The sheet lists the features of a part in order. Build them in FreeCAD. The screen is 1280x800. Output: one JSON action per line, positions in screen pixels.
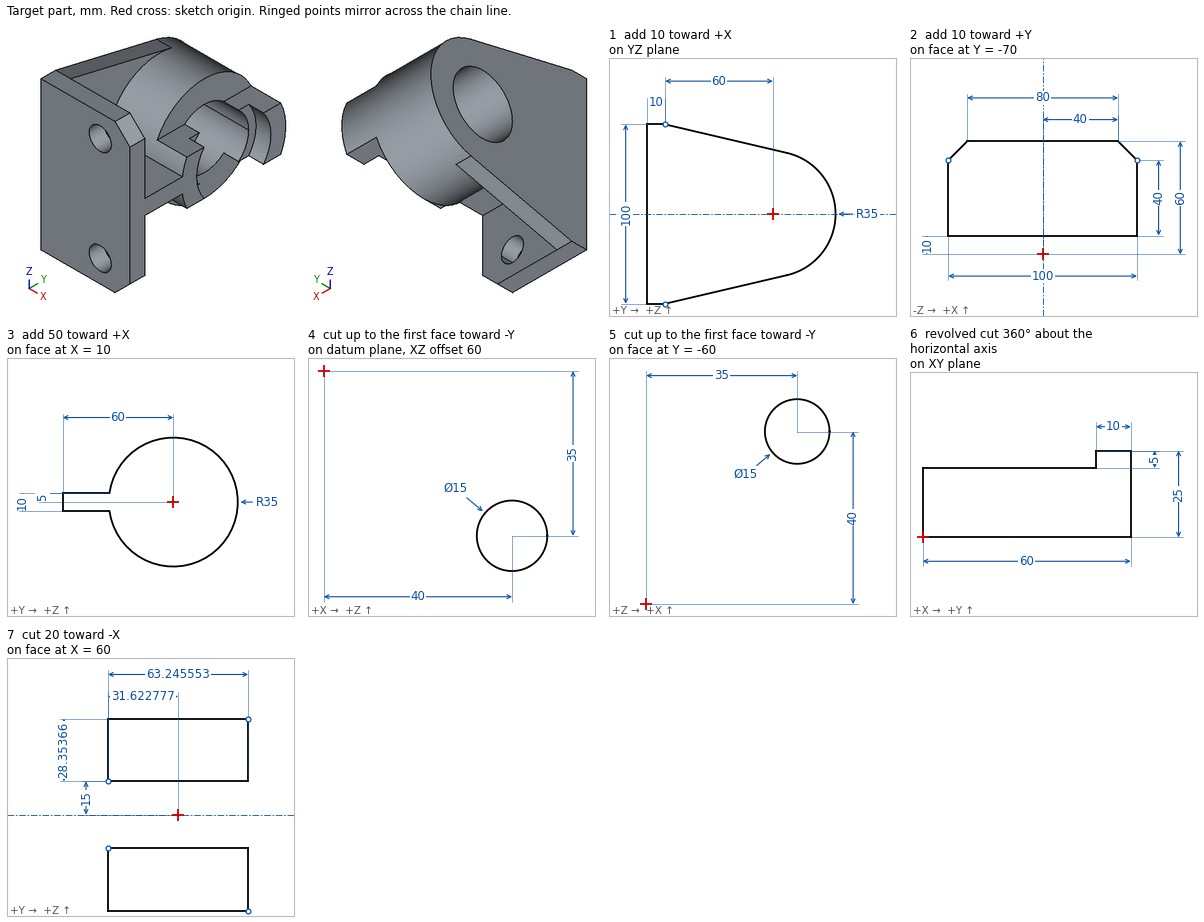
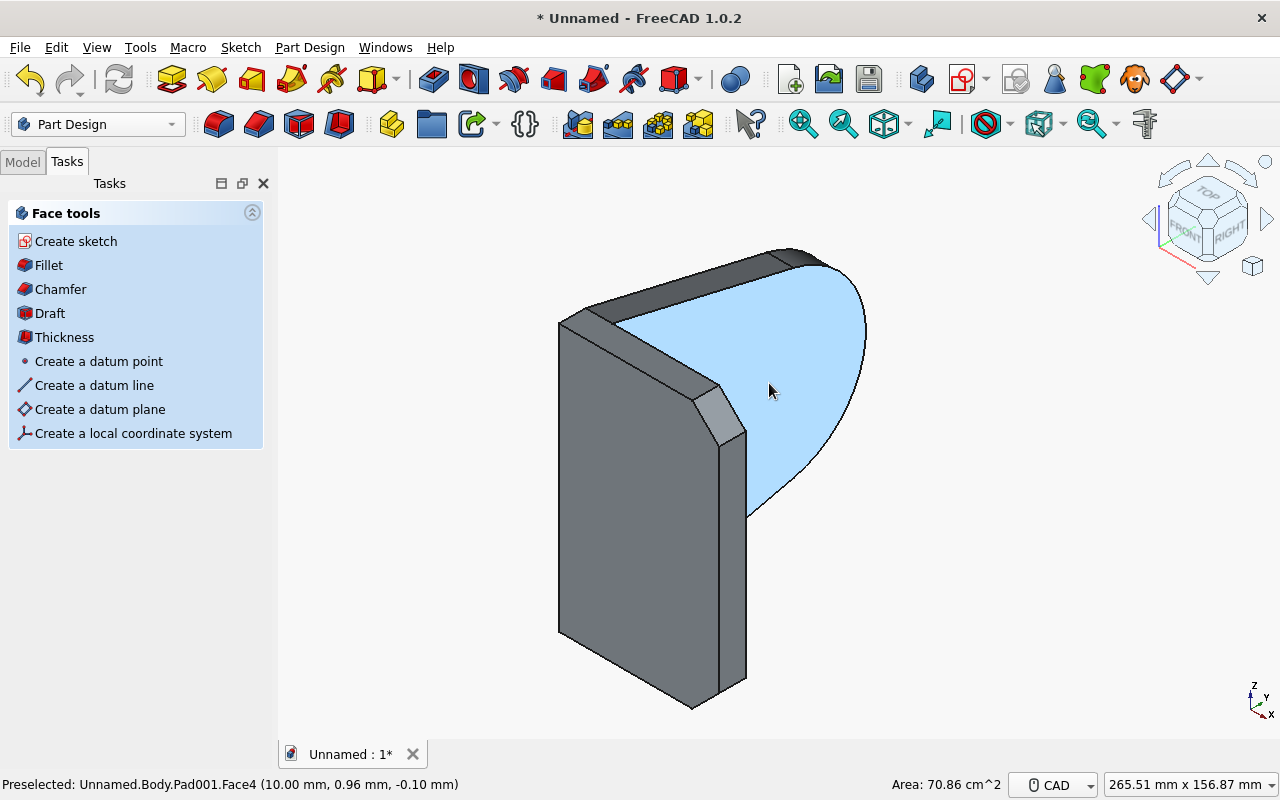
{"action": "left_click", "coordinate": [962, 80]}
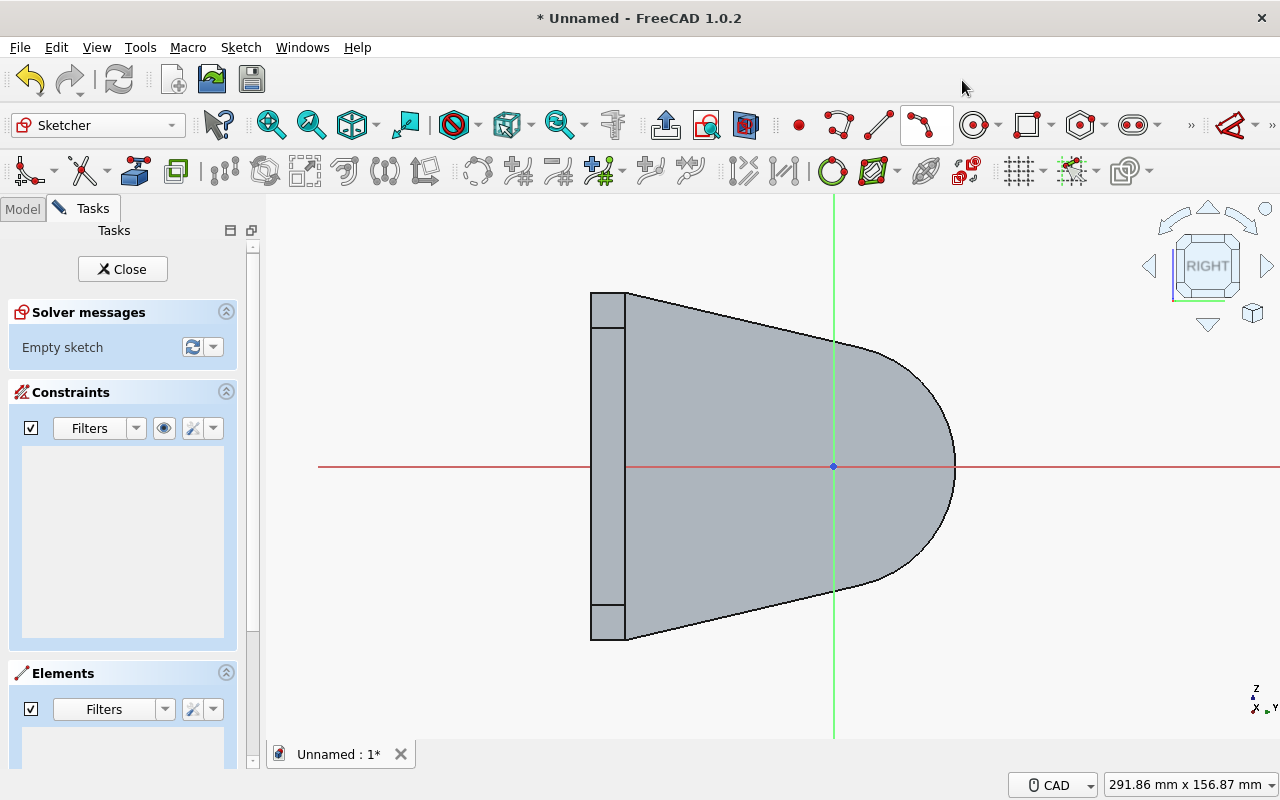
{"action": "left_click", "coordinate": [746, 126]}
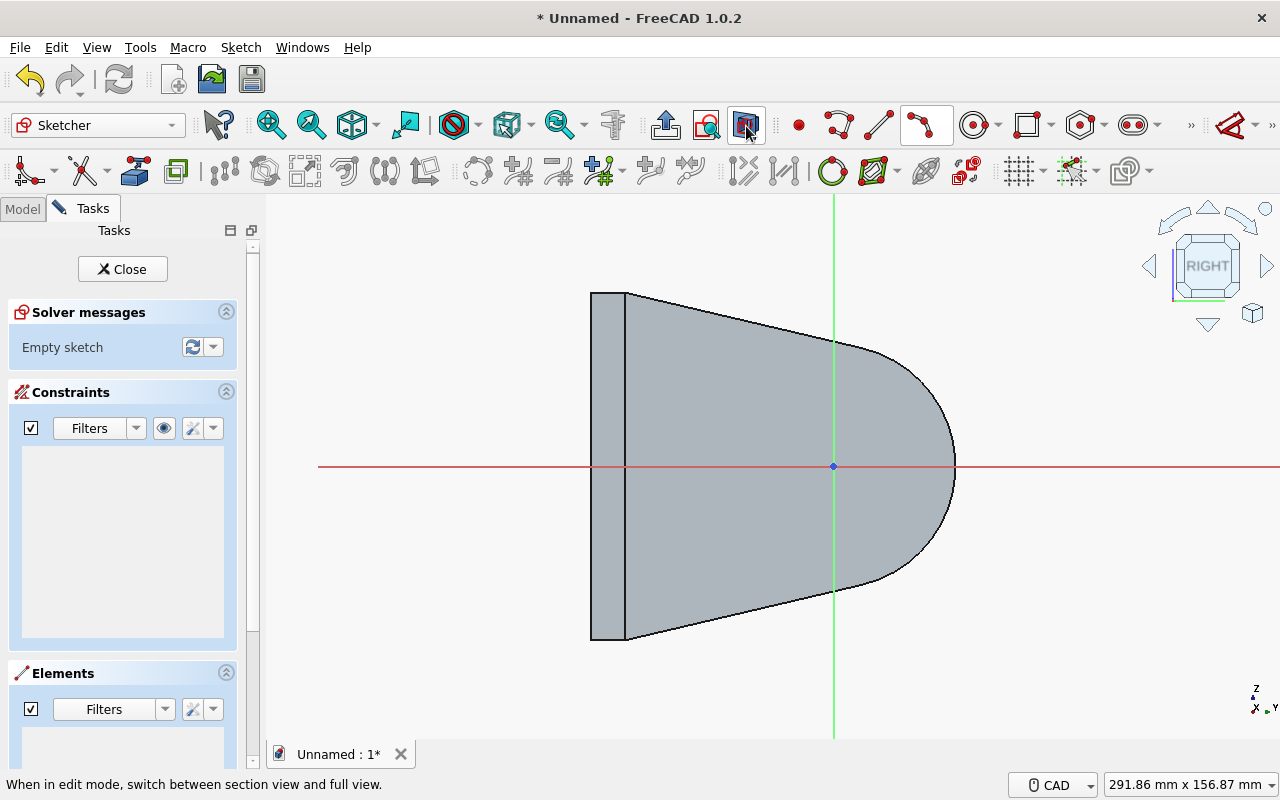
{"action": "scroll", "coordinate": [895, 466], "scroll_direction": "up", "scroll_amount": 3}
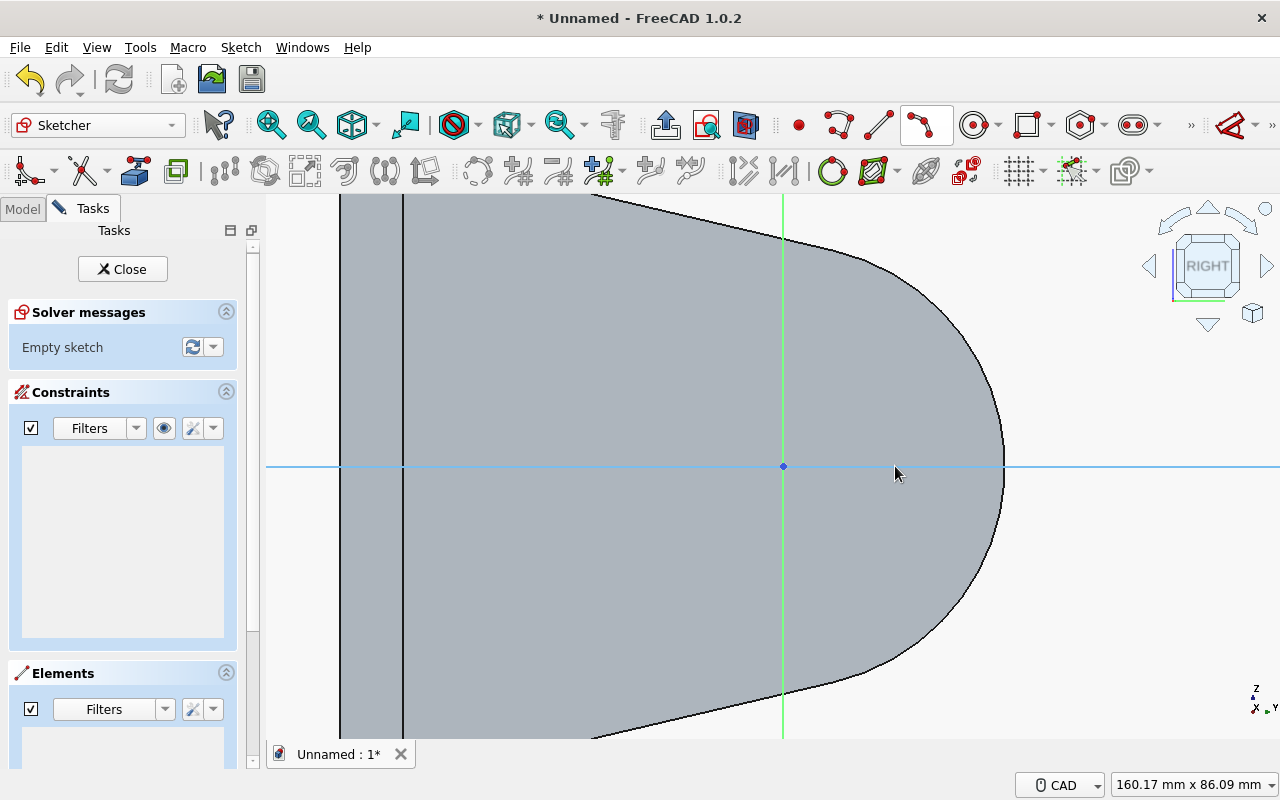
{"action": "left_click", "coordinate": [840, 126]}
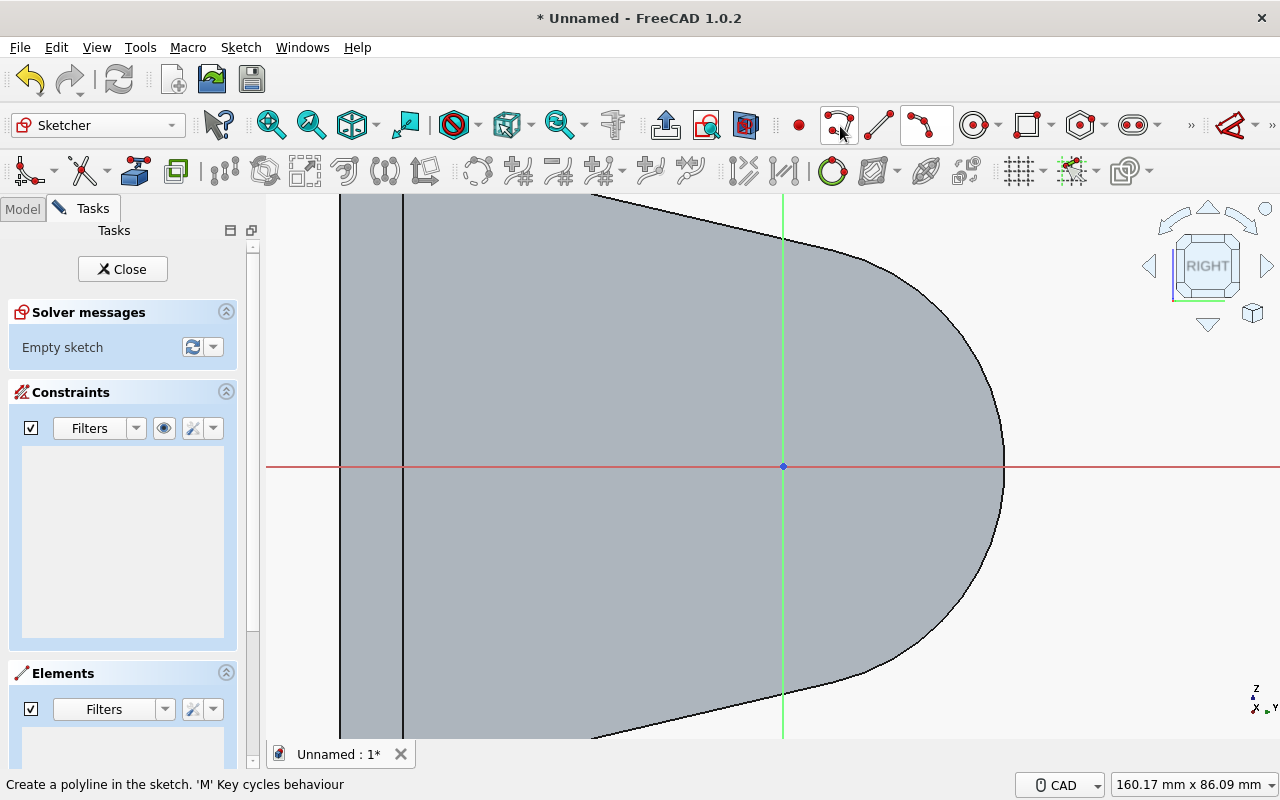
{"action": "left_click", "coordinate": [564, 435]}
{"action": "left_click", "coordinate": [403, 435]}
{"action": "left_click", "coordinate": [403, 498]}
{"action": "left_click", "coordinate": [564, 498]}
{"action": "right_click", "coordinate": [564, 498]}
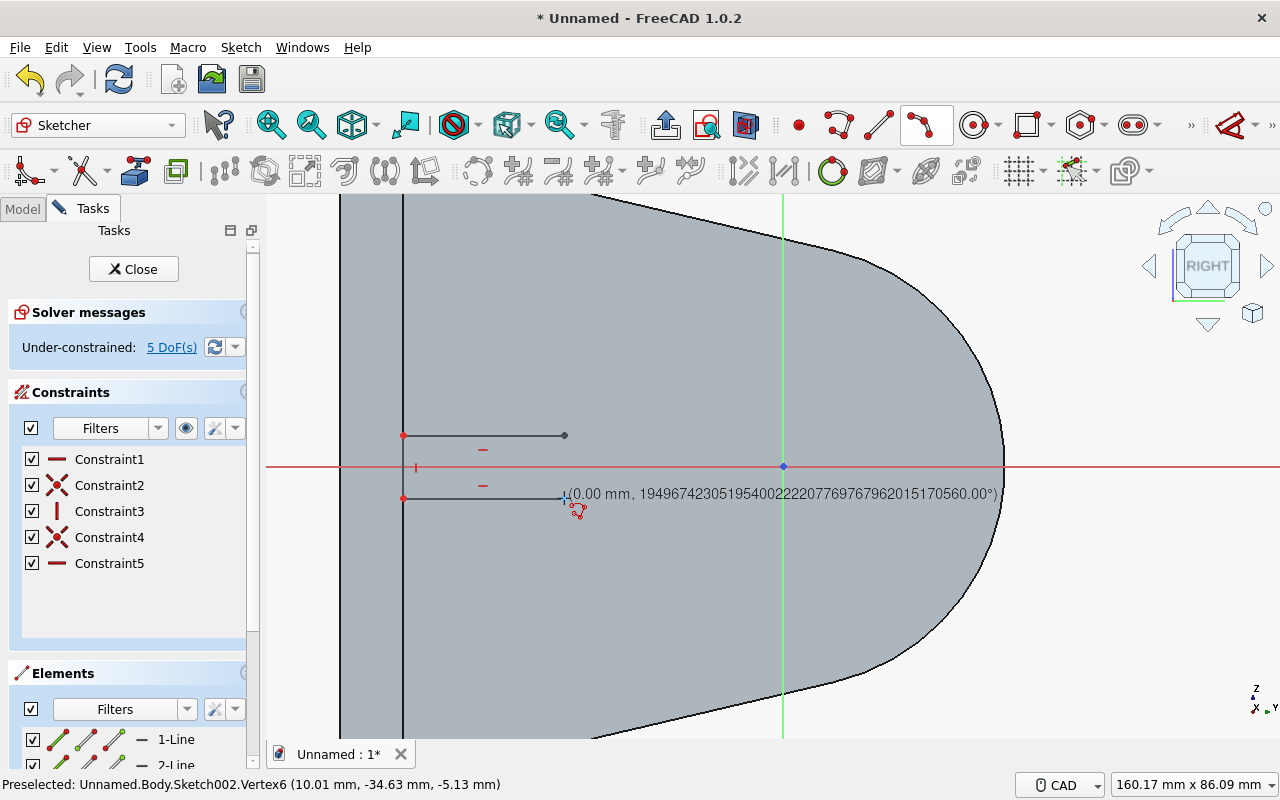
{"action": "left_click", "coordinate": [920, 126]}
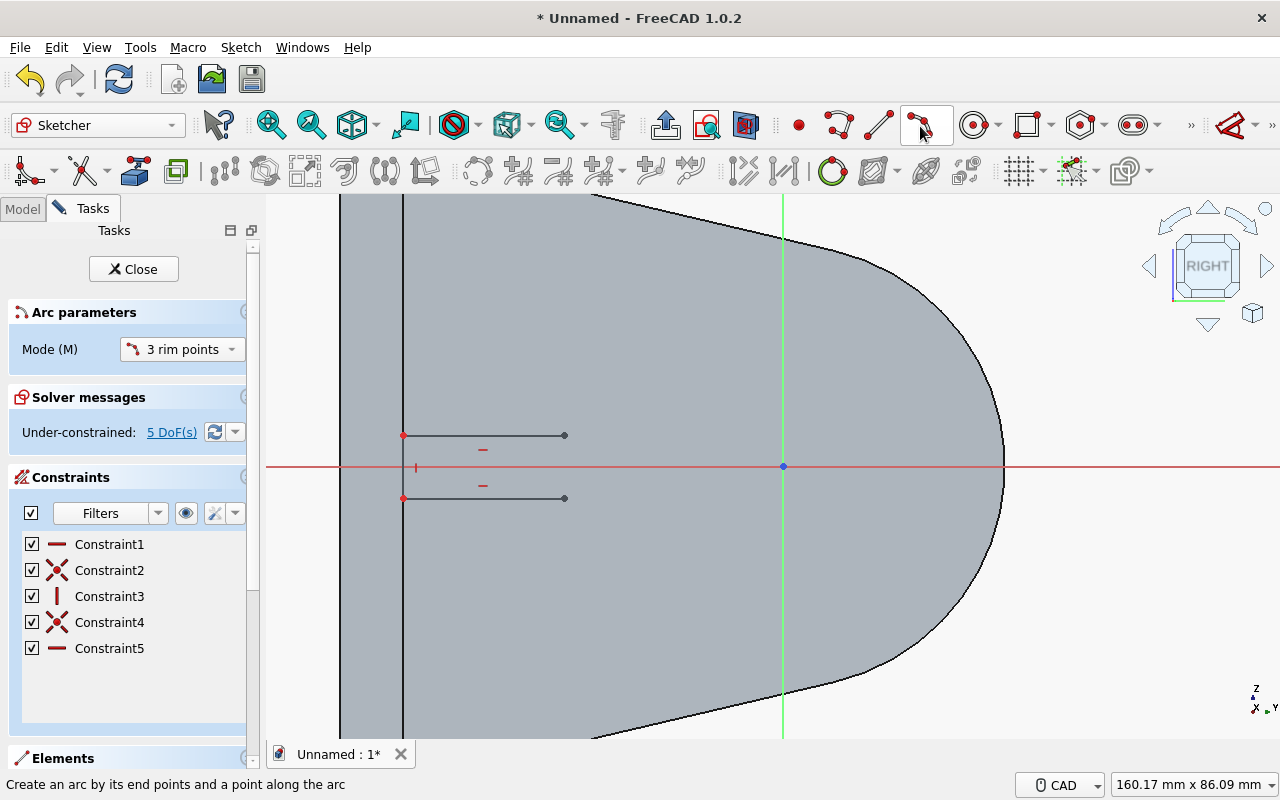
{"action": "left_click", "coordinate": [564, 499]}
{"action": "left_click", "coordinate": [564, 436]}
{"action": "left_click", "coordinate": [966, 592]}
{"action": "key", "text": "Escape"}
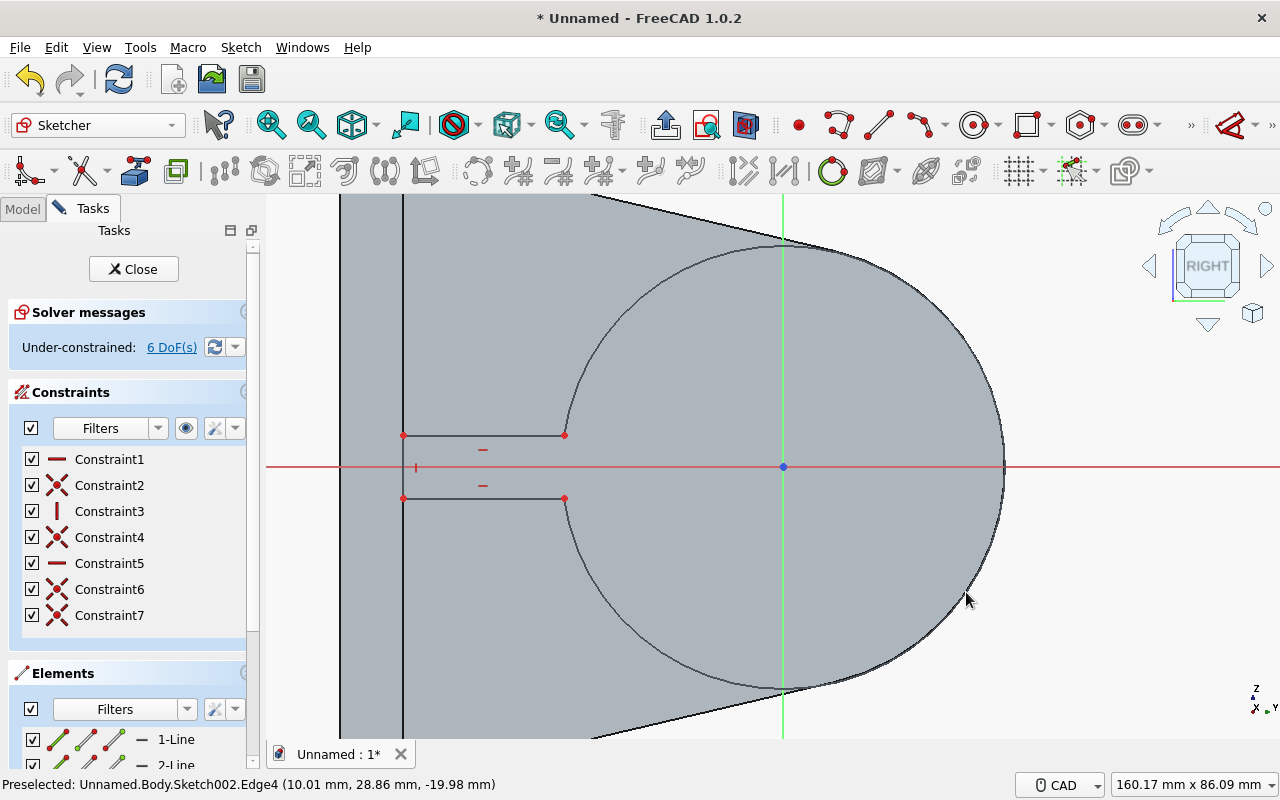
{"action": "left_click_drag", "start_coordinate": [773, 456], "coordinate": [793, 478]}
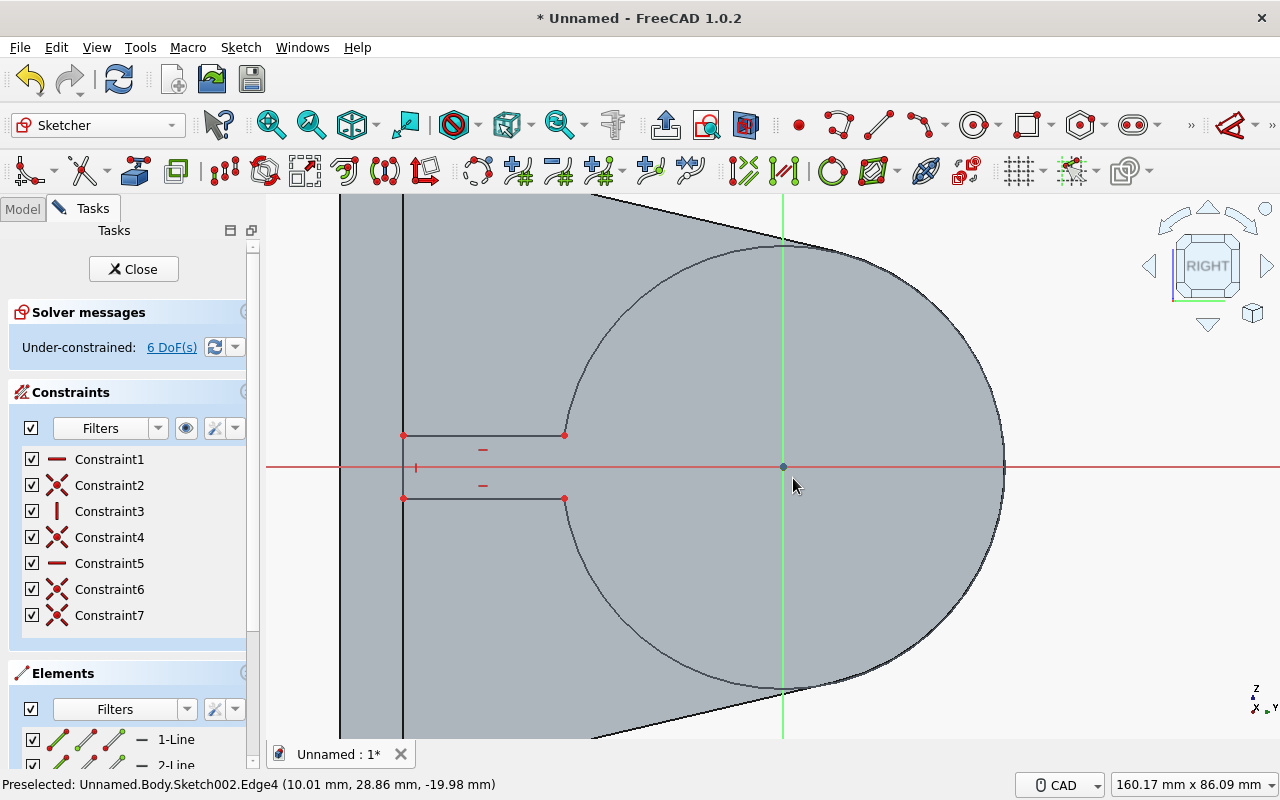
{"action": "key", "text": "c"}